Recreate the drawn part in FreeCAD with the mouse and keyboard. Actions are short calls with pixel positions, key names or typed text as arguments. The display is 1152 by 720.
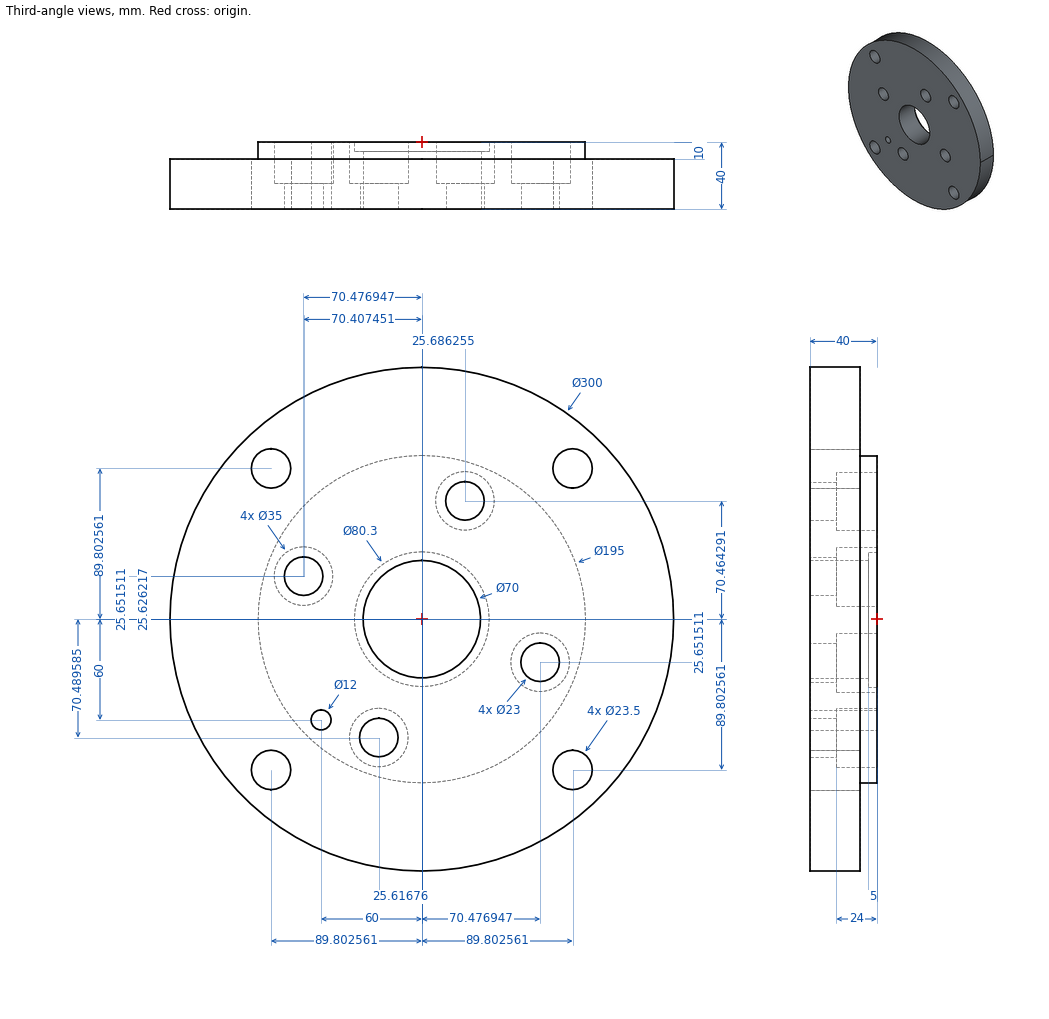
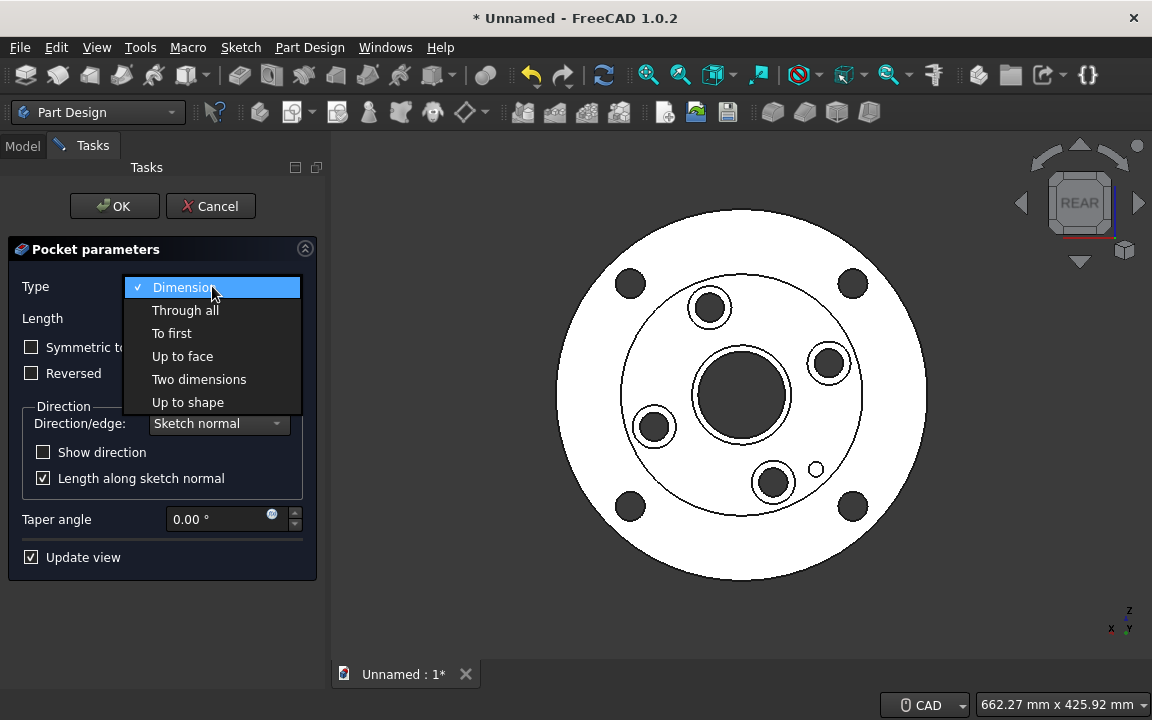
click(212, 310)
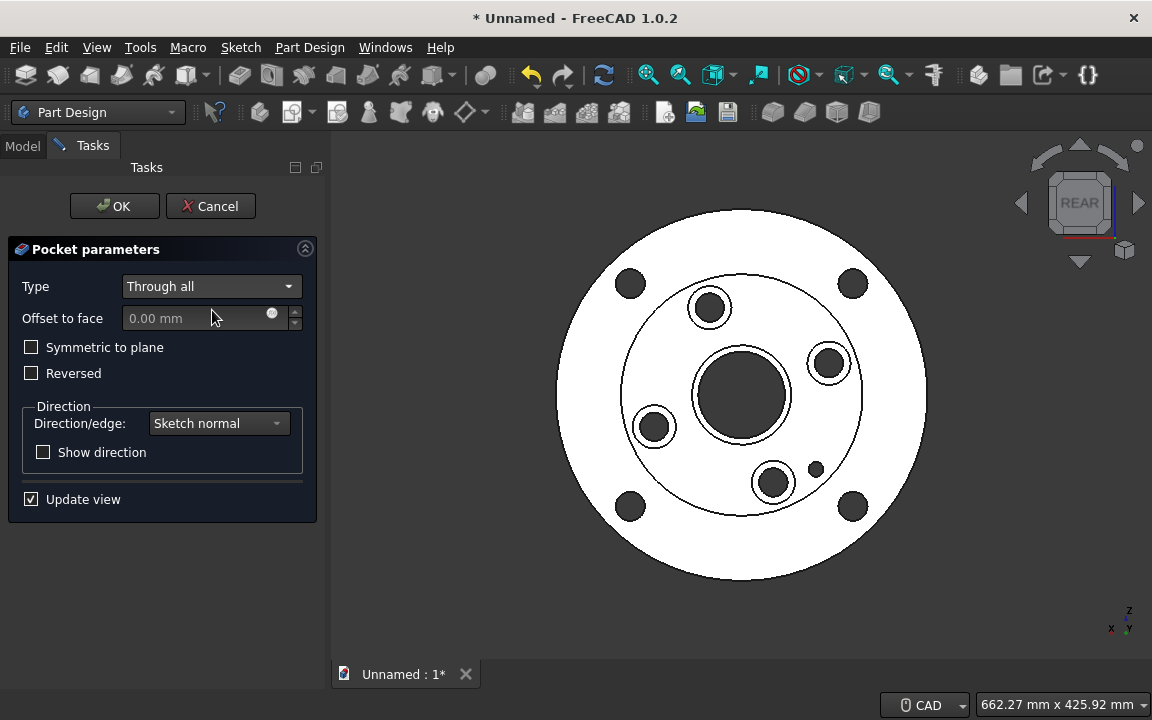
click(115, 206)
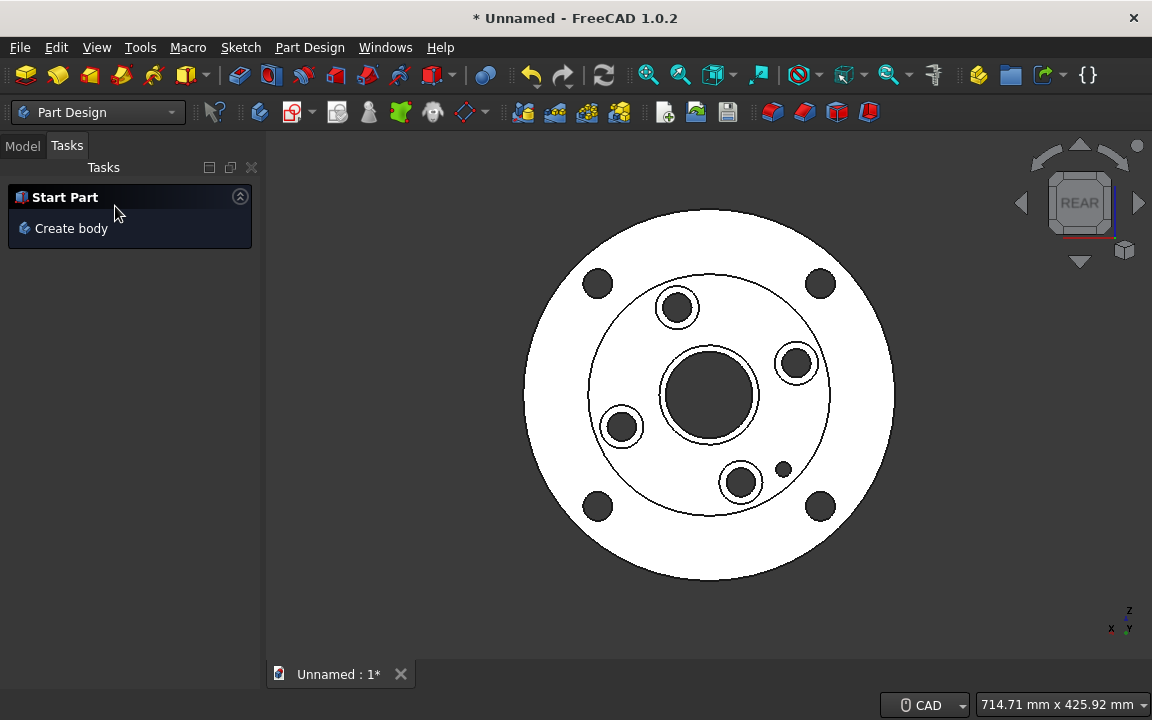
key(0)